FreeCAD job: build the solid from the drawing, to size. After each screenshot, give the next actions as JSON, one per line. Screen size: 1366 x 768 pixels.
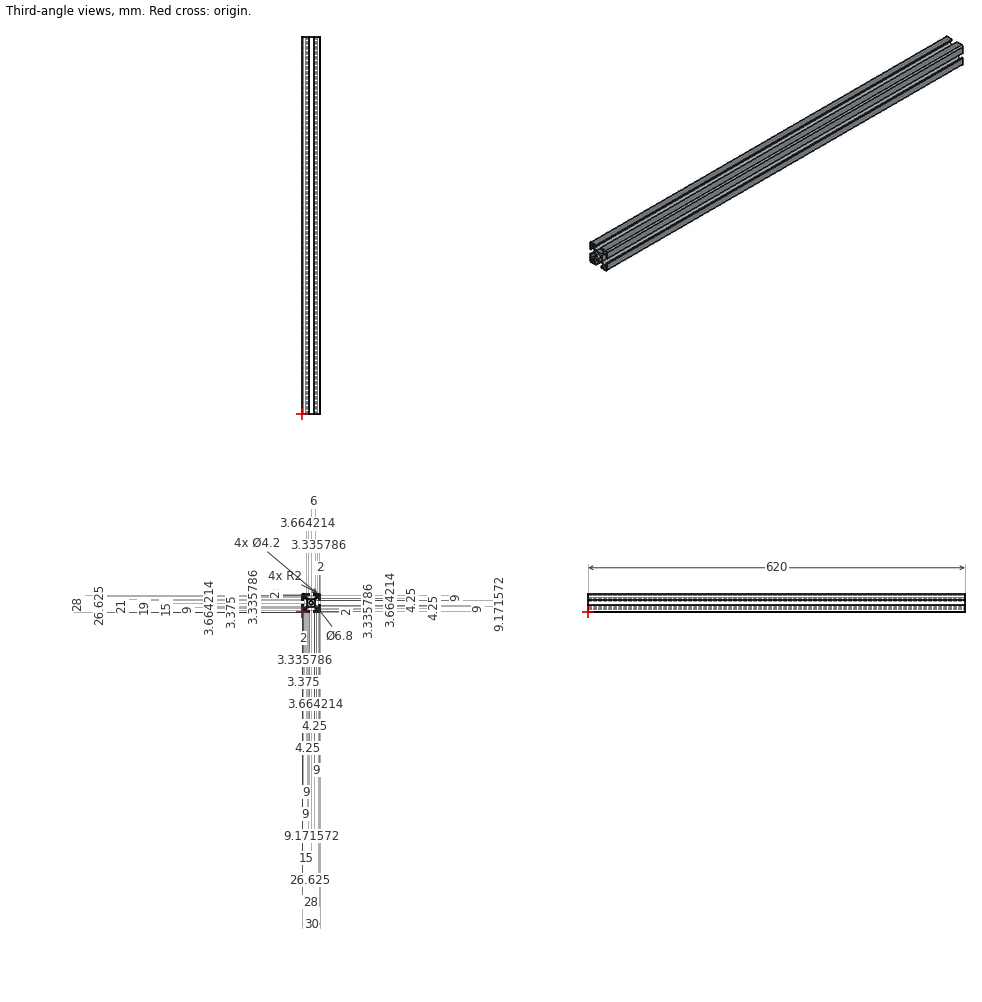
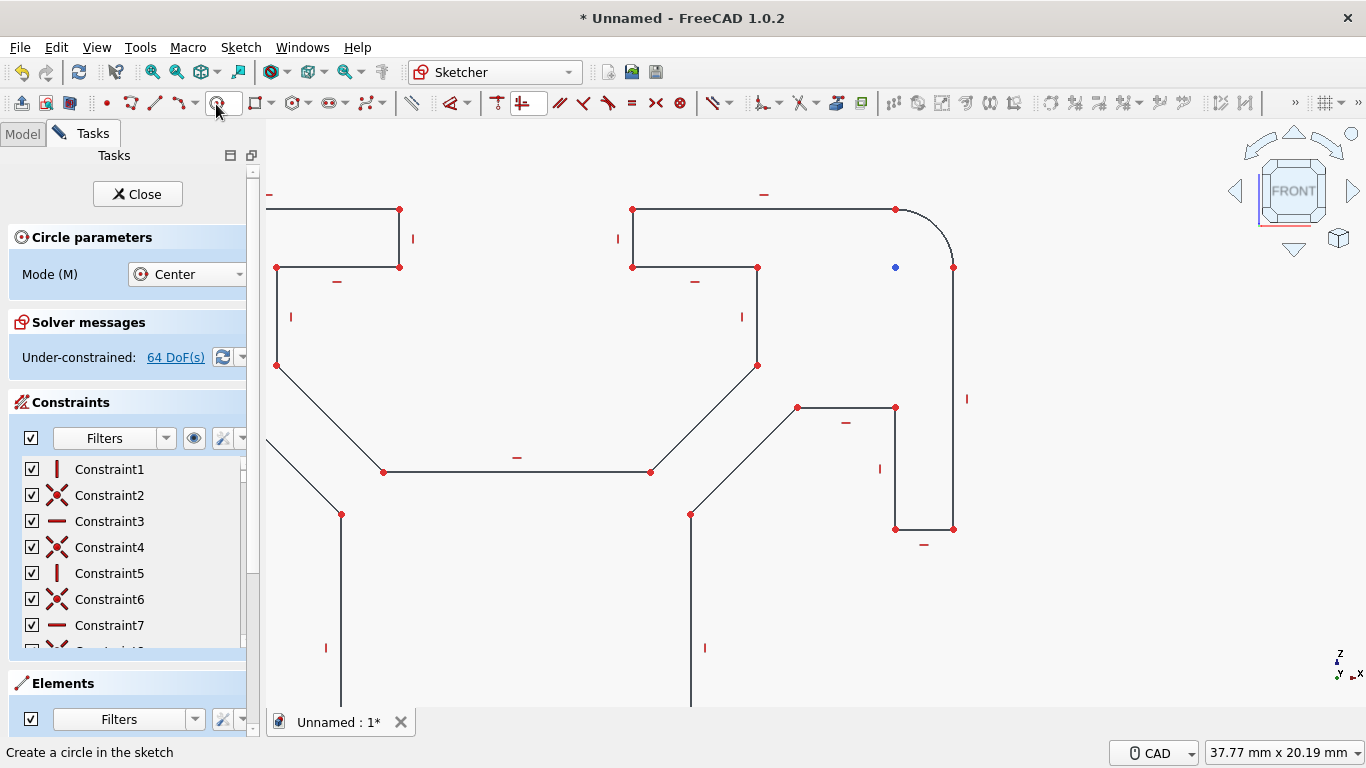
{"action": "left_click", "coordinate": [855, 306]}
{"action": "left_click", "coordinate": [812, 263]}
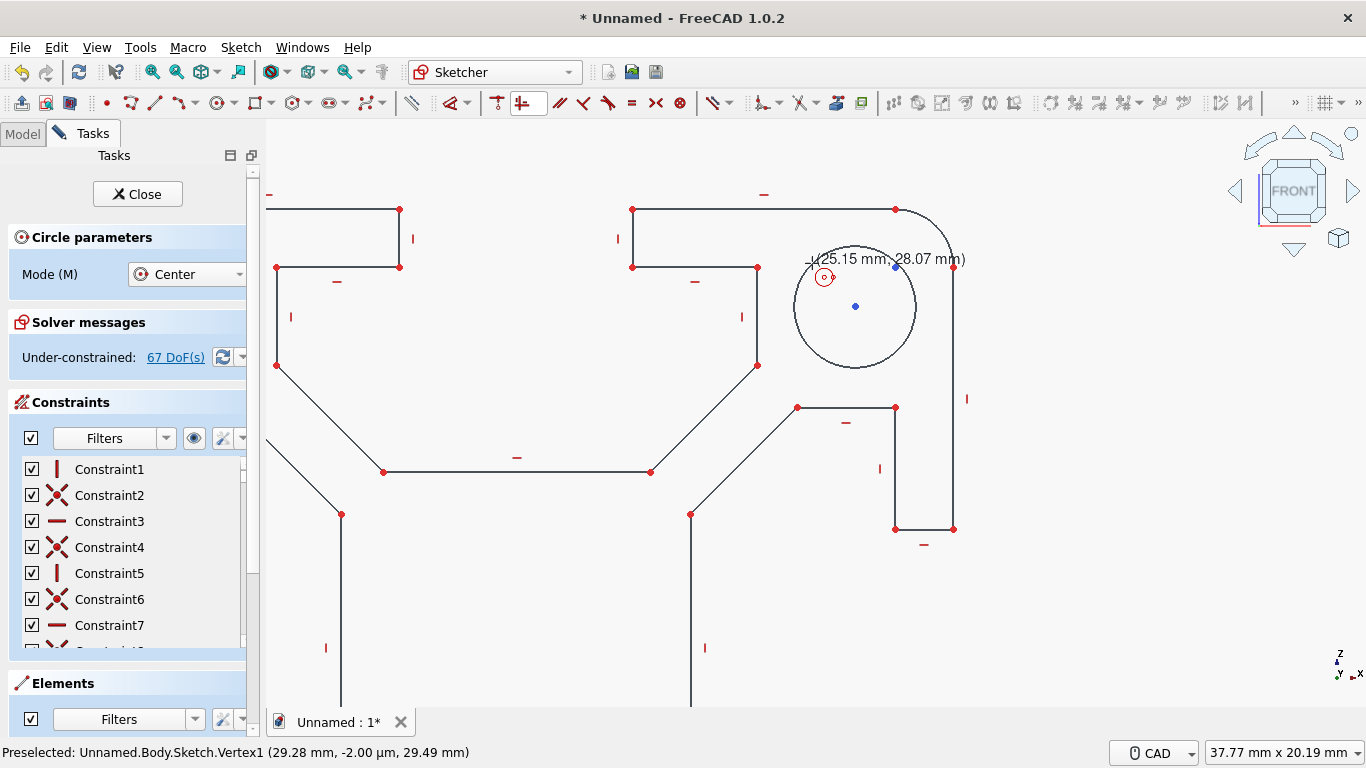
{"action": "scroll", "coordinate": [936, 224], "scroll_direction": "down", "scroll_amount": 4}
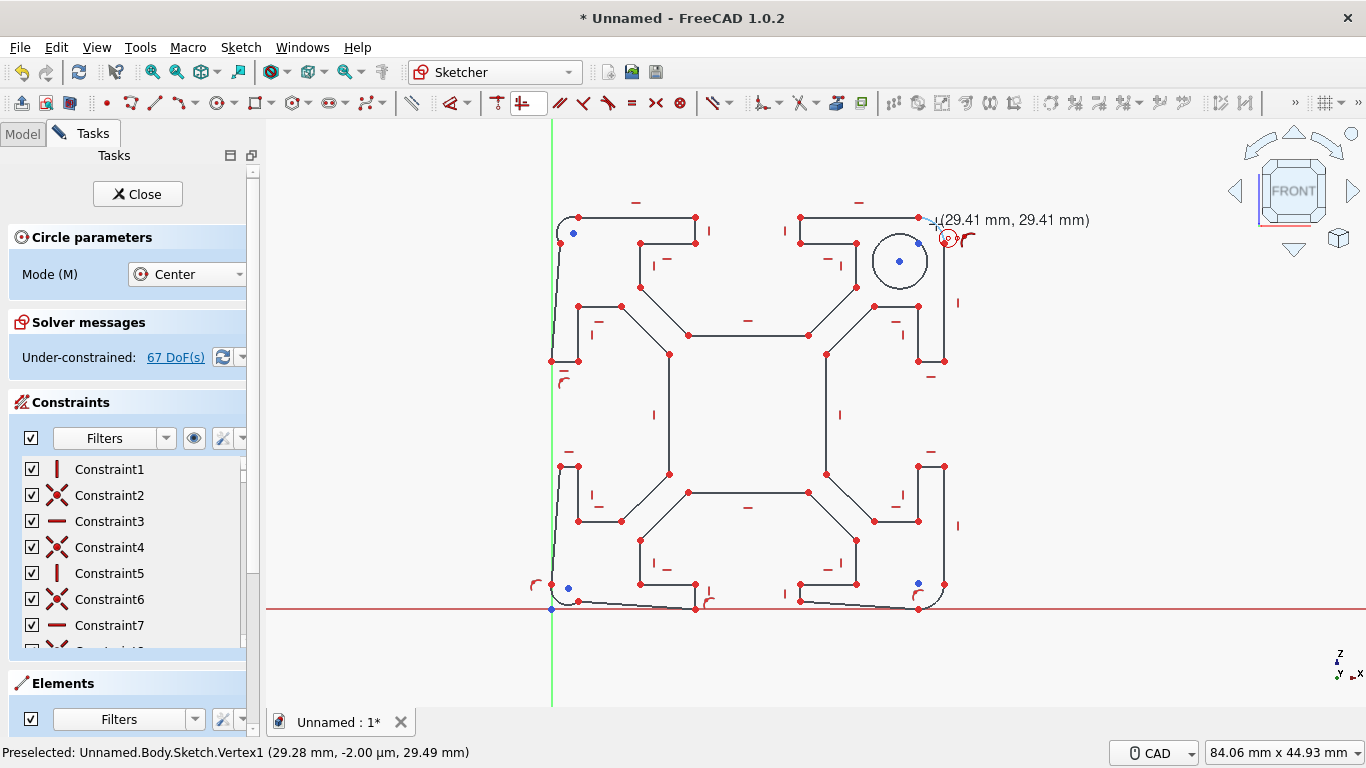
{"action": "left_click", "coordinate": [596, 261]}
{"action": "left_click", "coordinate": [615, 242]}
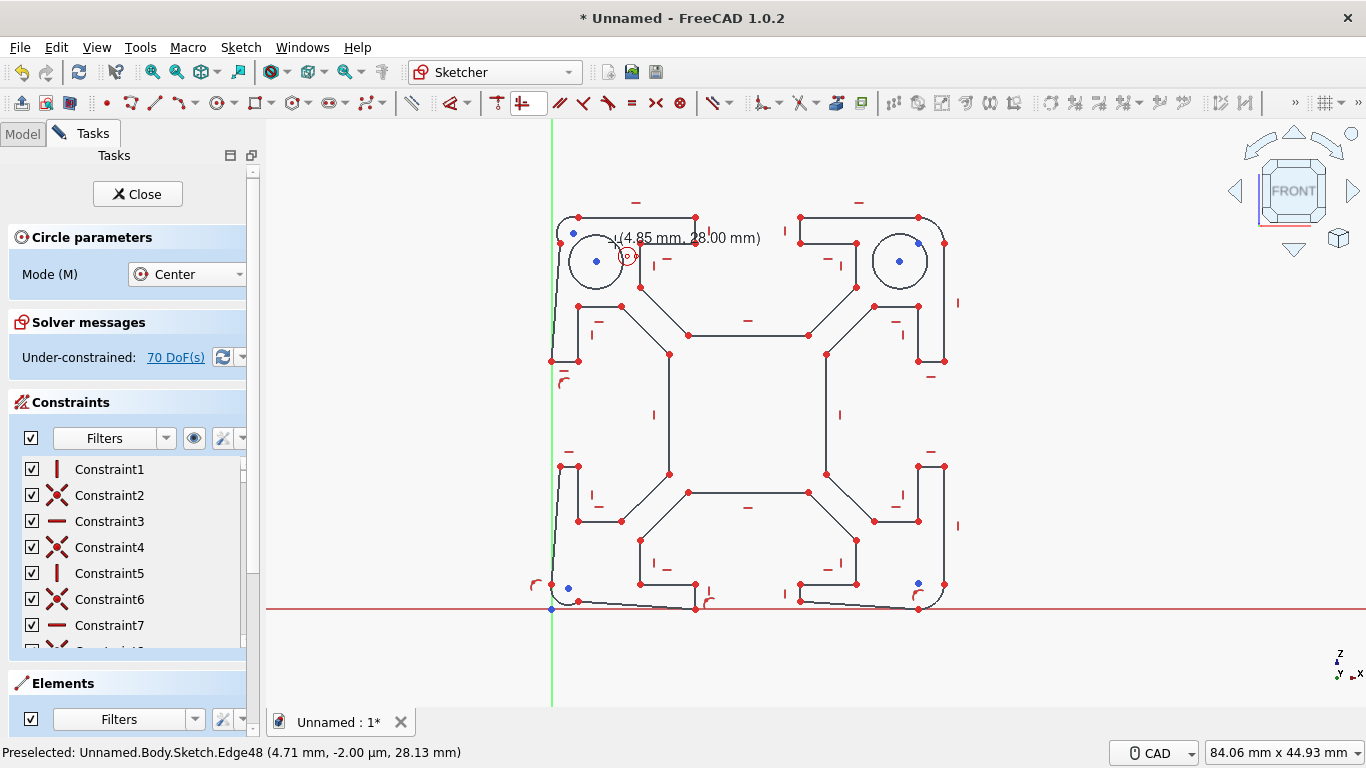
{"action": "left_click", "coordinate": [900, 565]}
{"action": "left_click", "coordinate": [919, 546]}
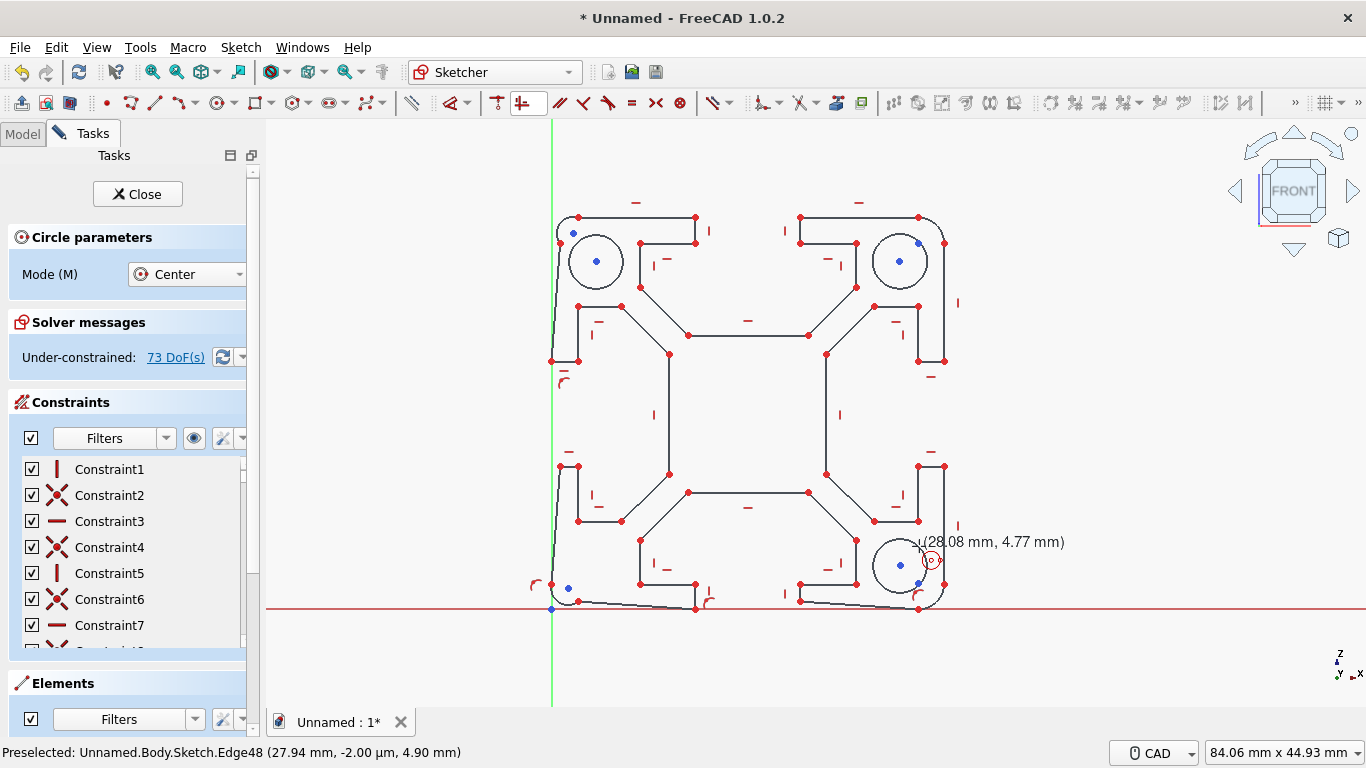
{"action": "left_click", "coordinate": [748, 413]}
{"action": "left_click", "coordinate": [779, 382]}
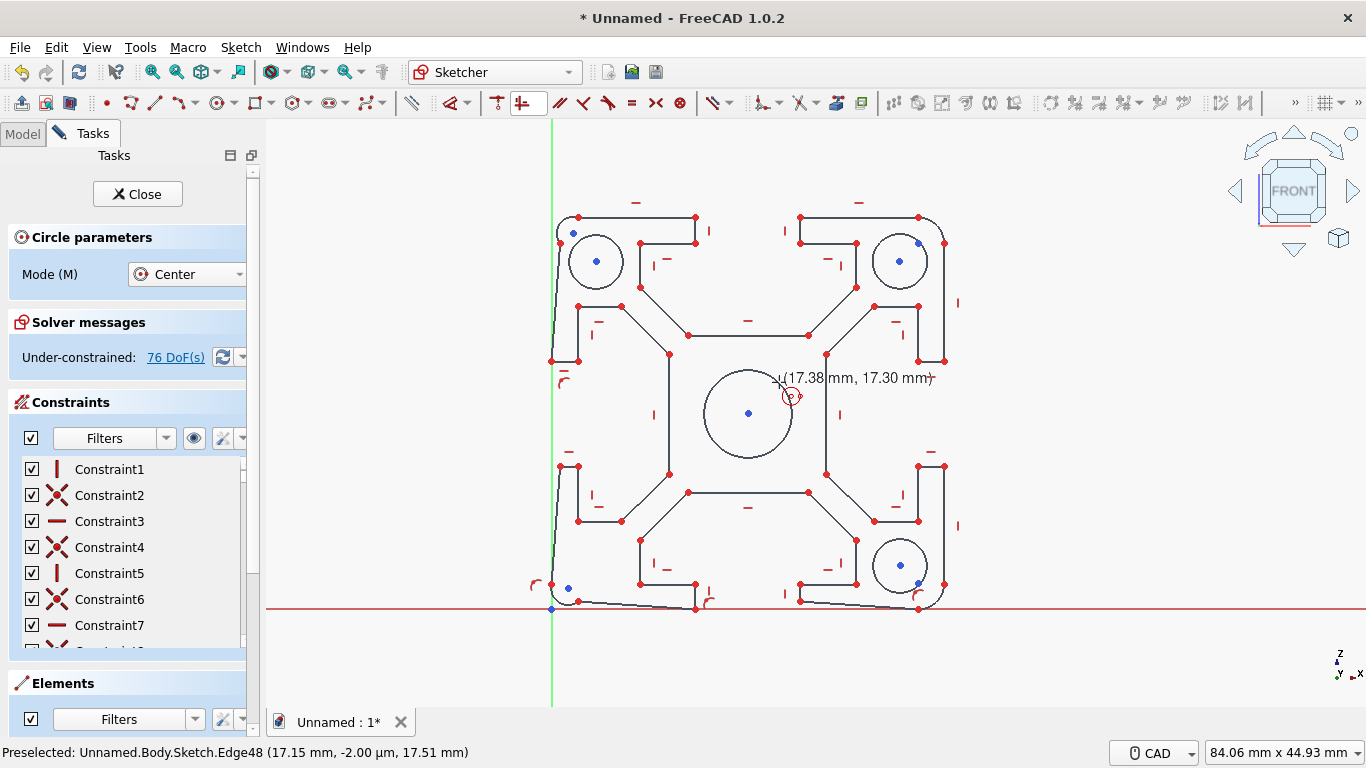
{"action": "left_click", "coordinate": [596, 565]}
{"action": "left_click", "coordinate": [615, 546]}
{"action": "key", "text": "Escape"}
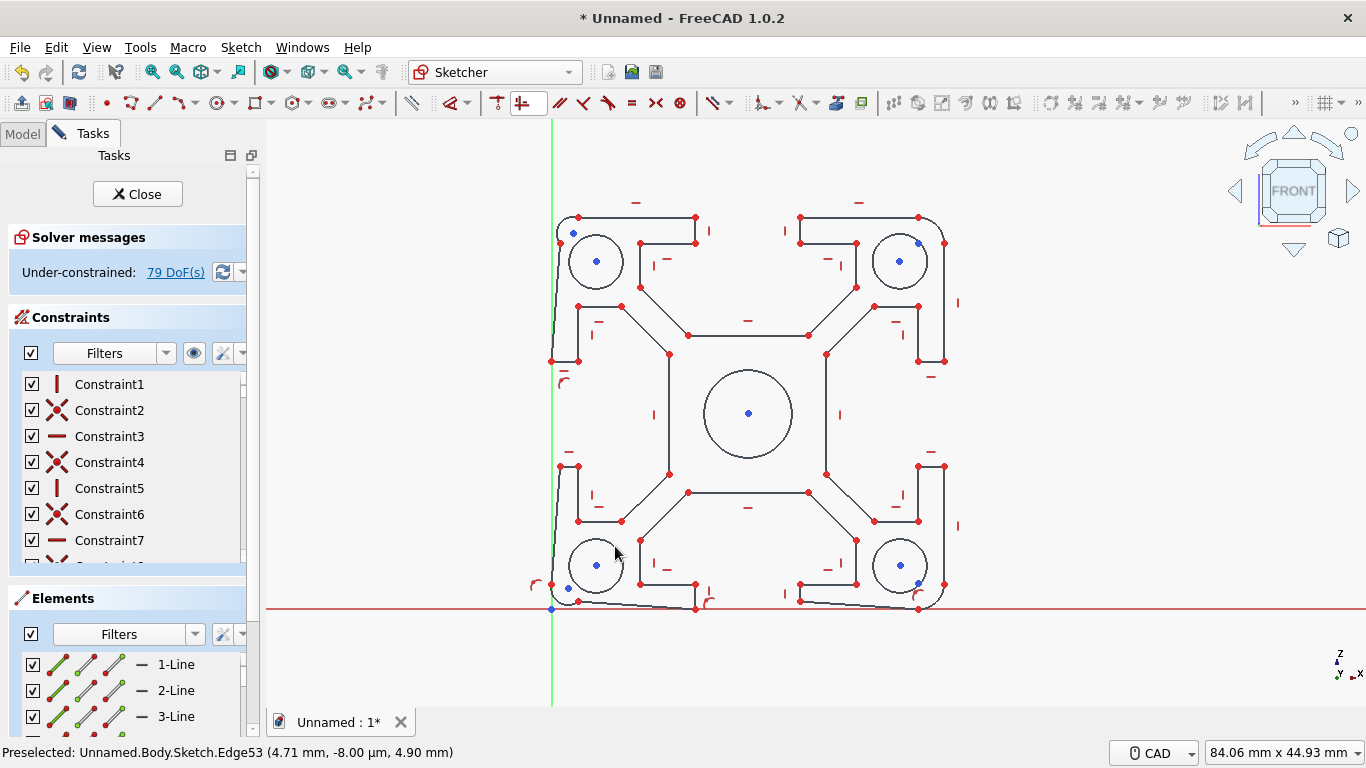
{"action": "left_click", "coordinate": [944, 279]}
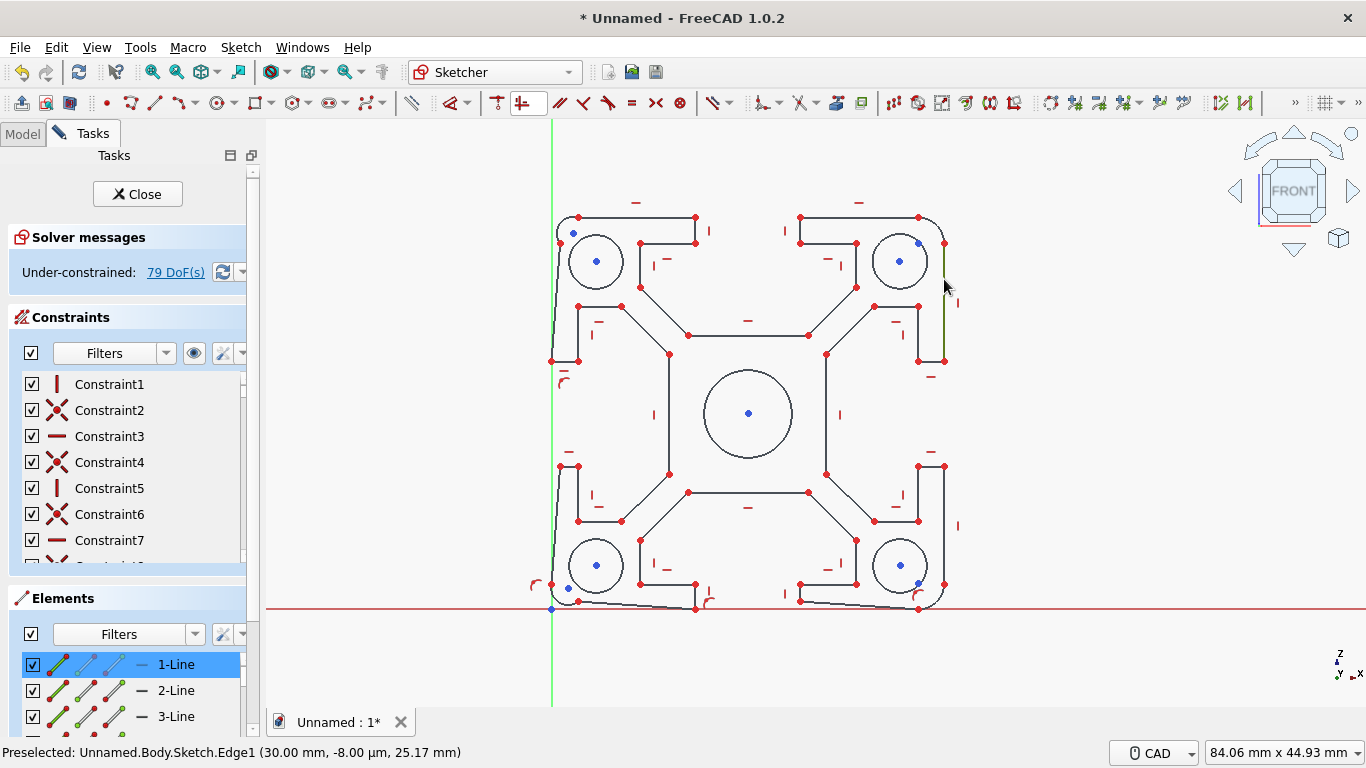
{"action": "left_click", "coordinate": [941, 232]}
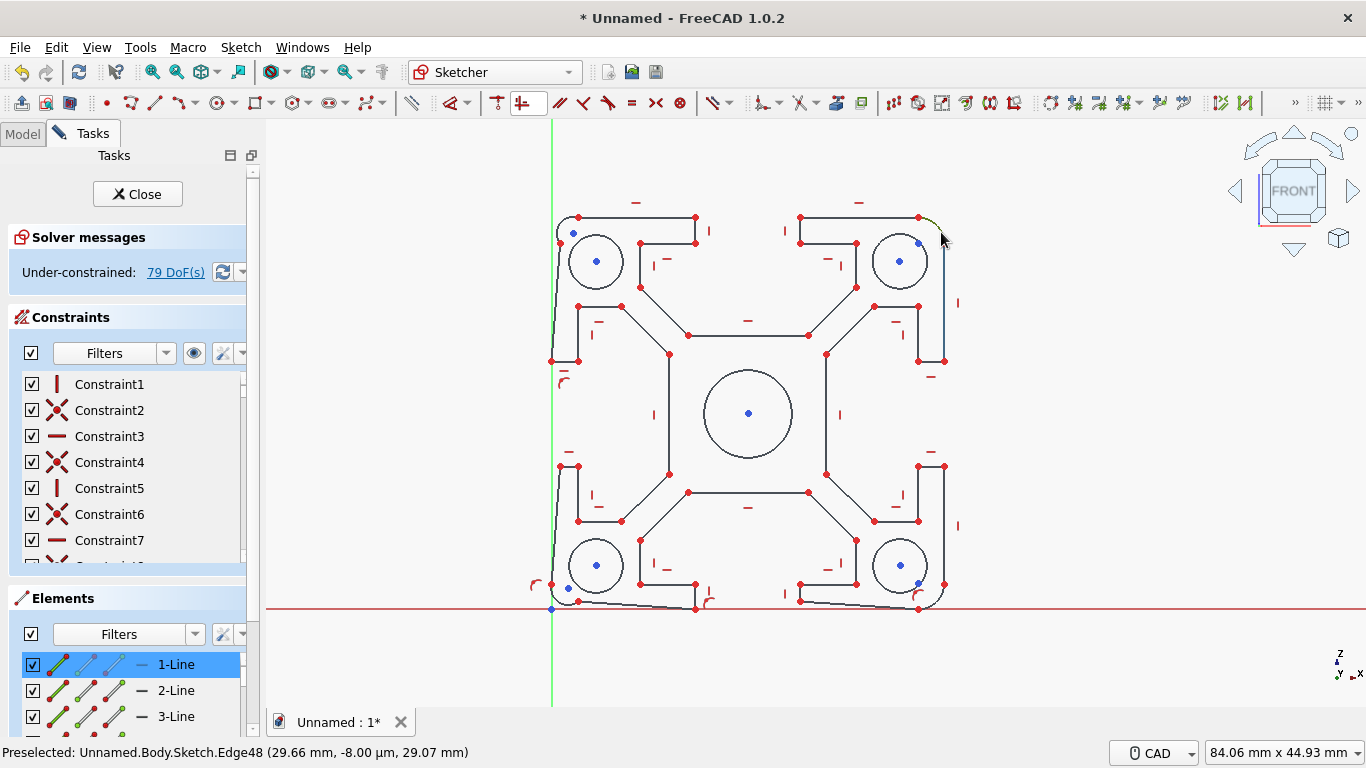
{"action": "key", "text": "t"}